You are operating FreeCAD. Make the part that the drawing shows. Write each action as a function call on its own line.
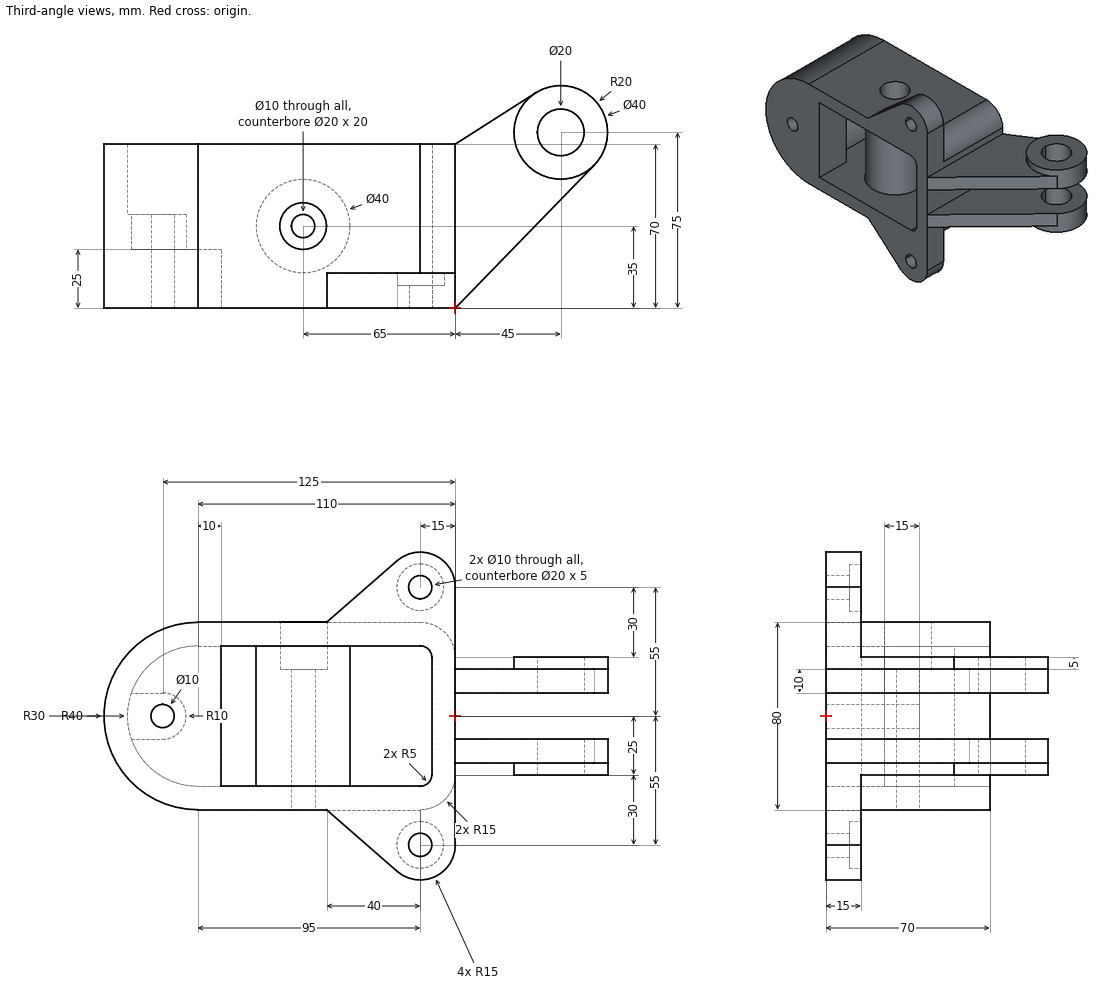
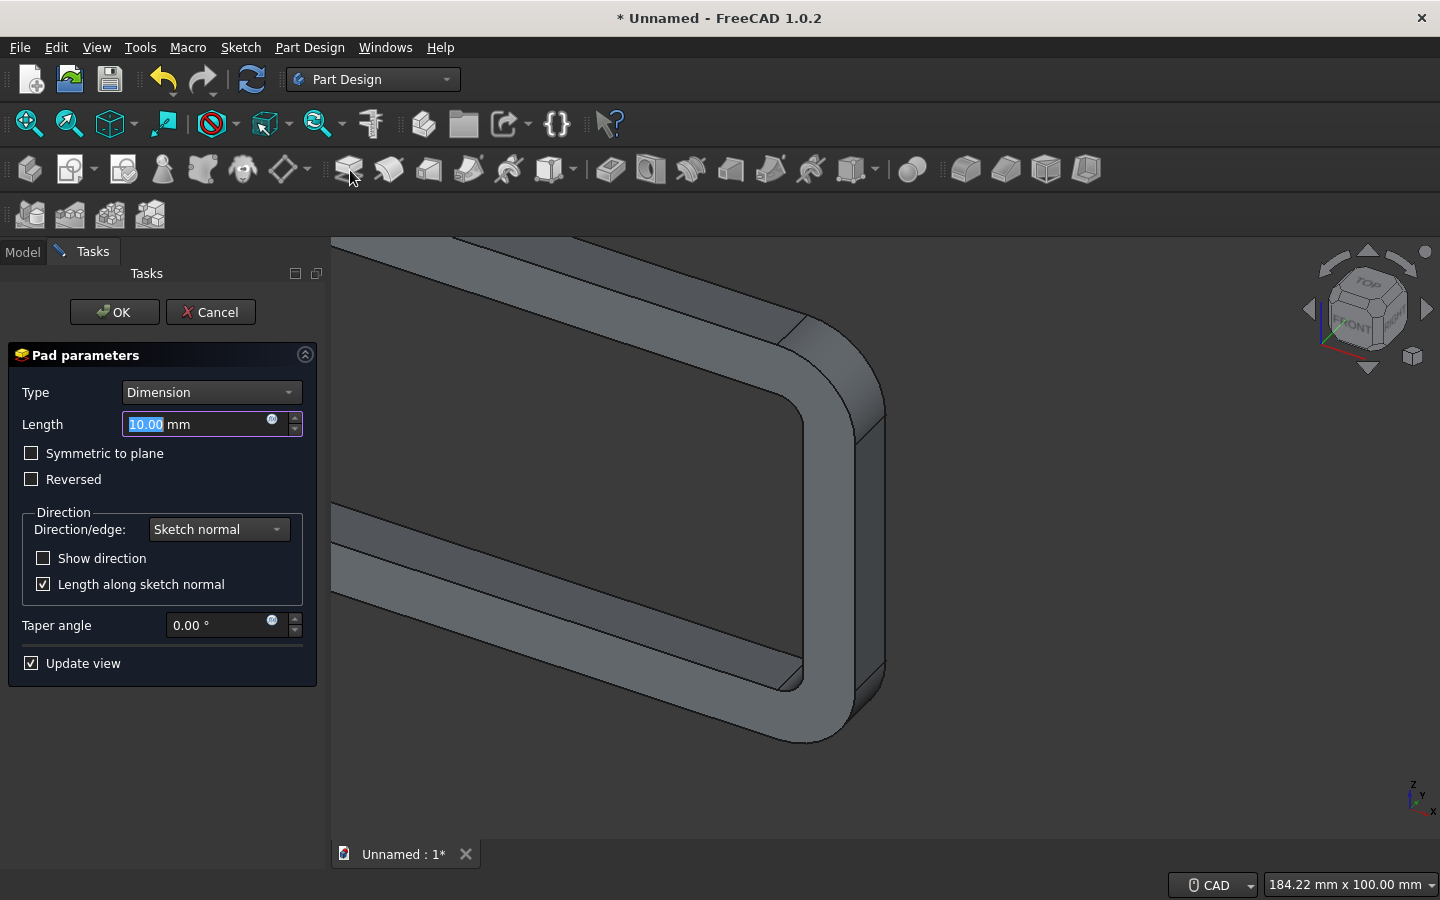
text(70)
key(Tab)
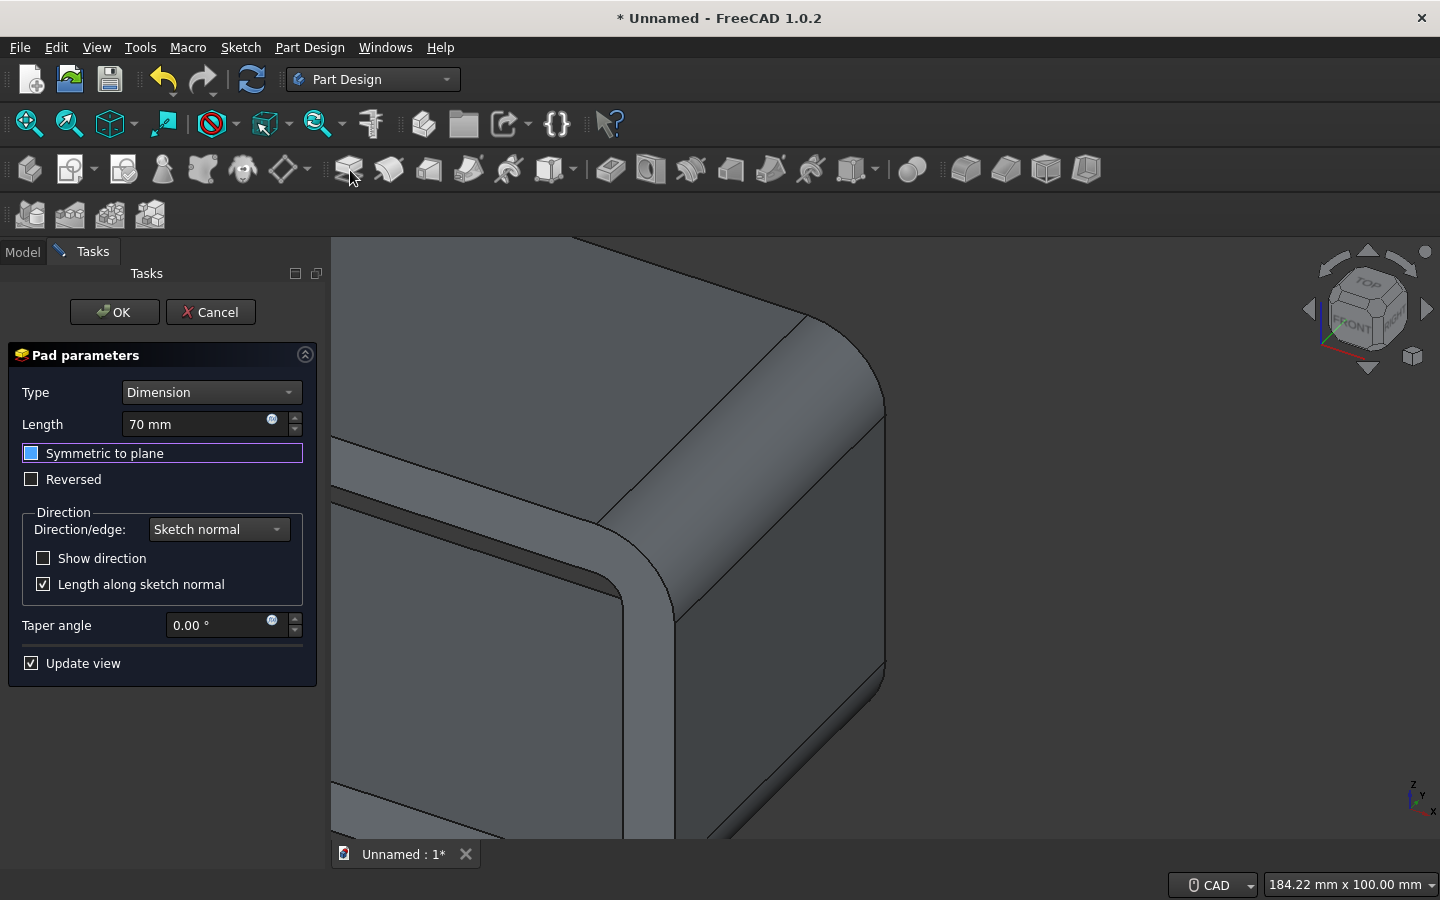
click(30, 479)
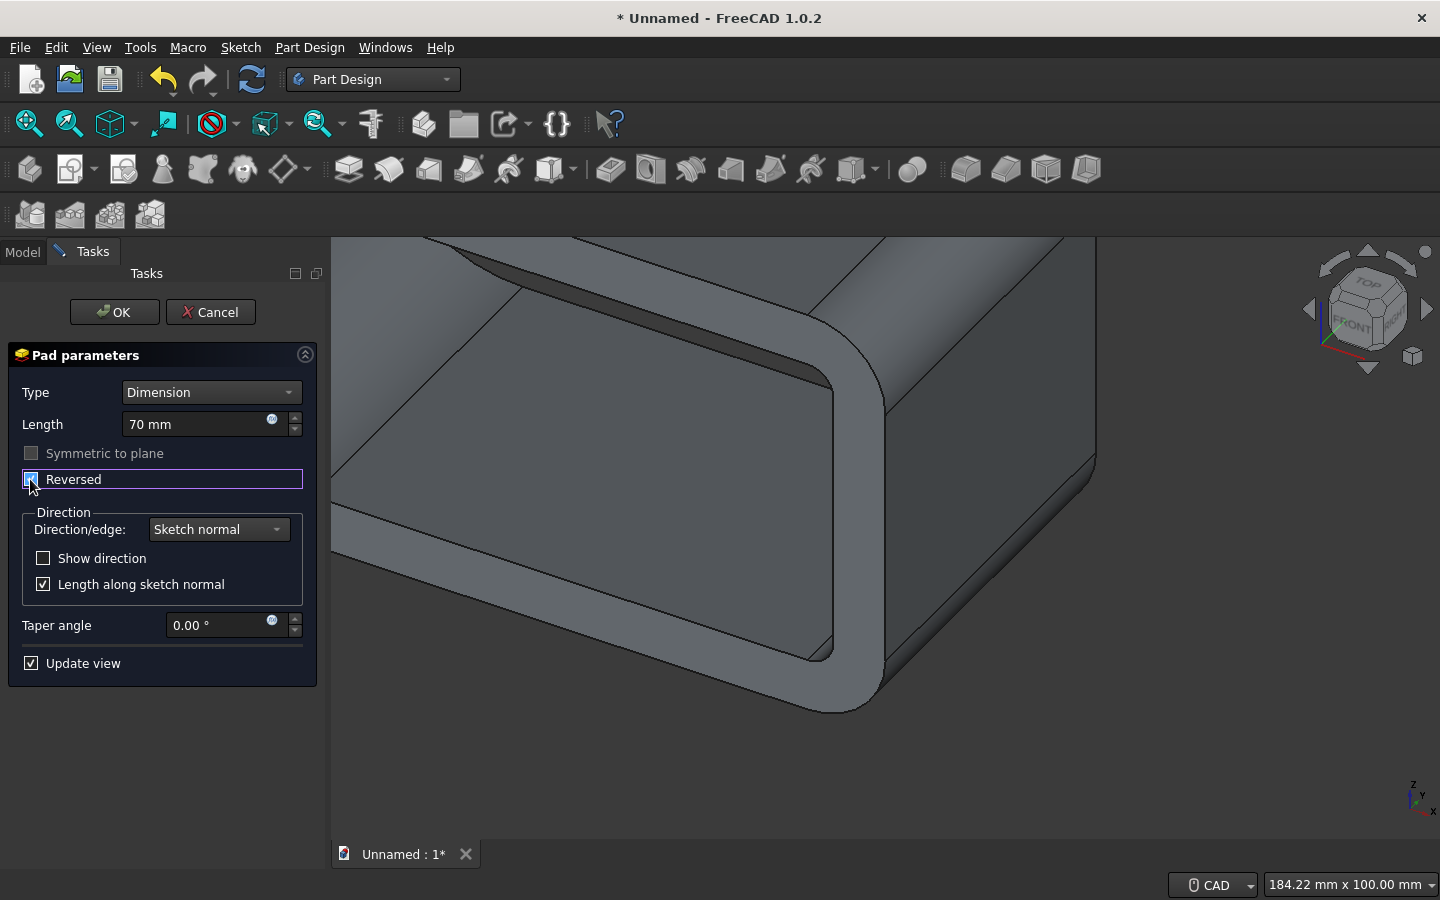
click(115, 312)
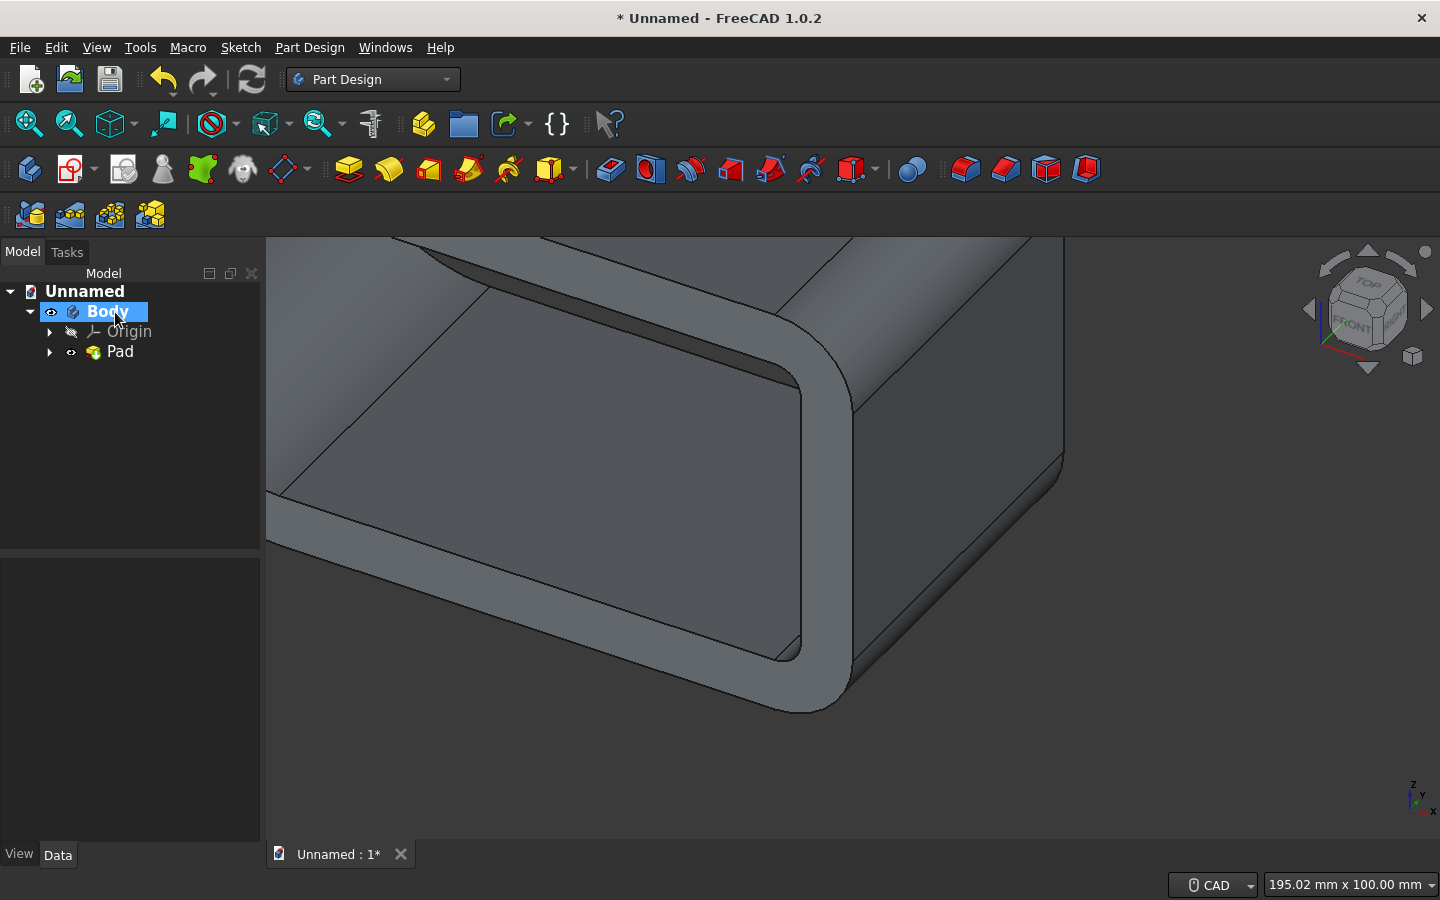
key(v)
key(f)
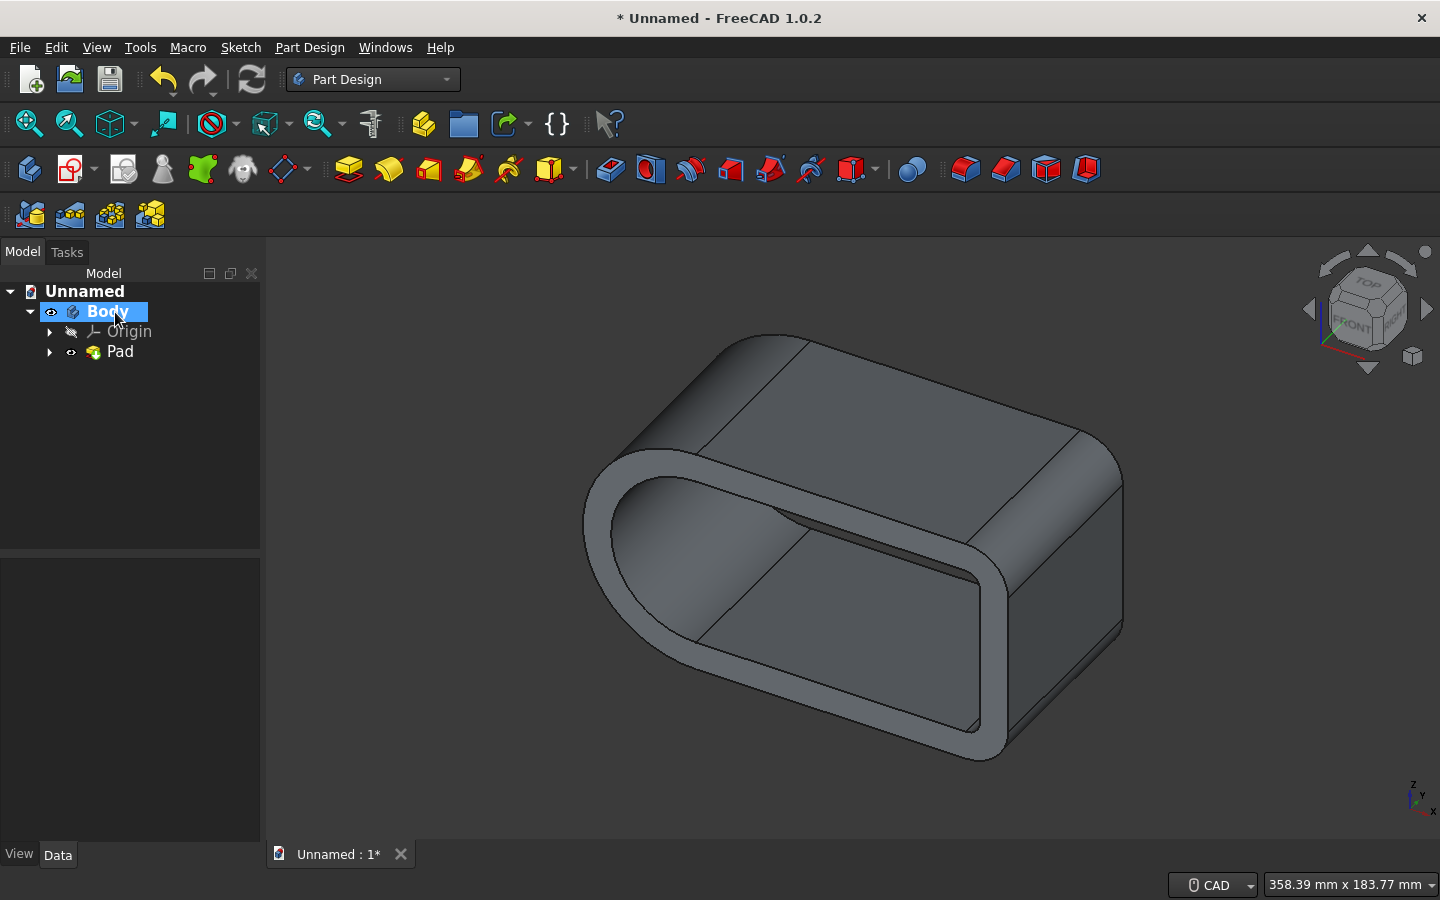
click(674, 646)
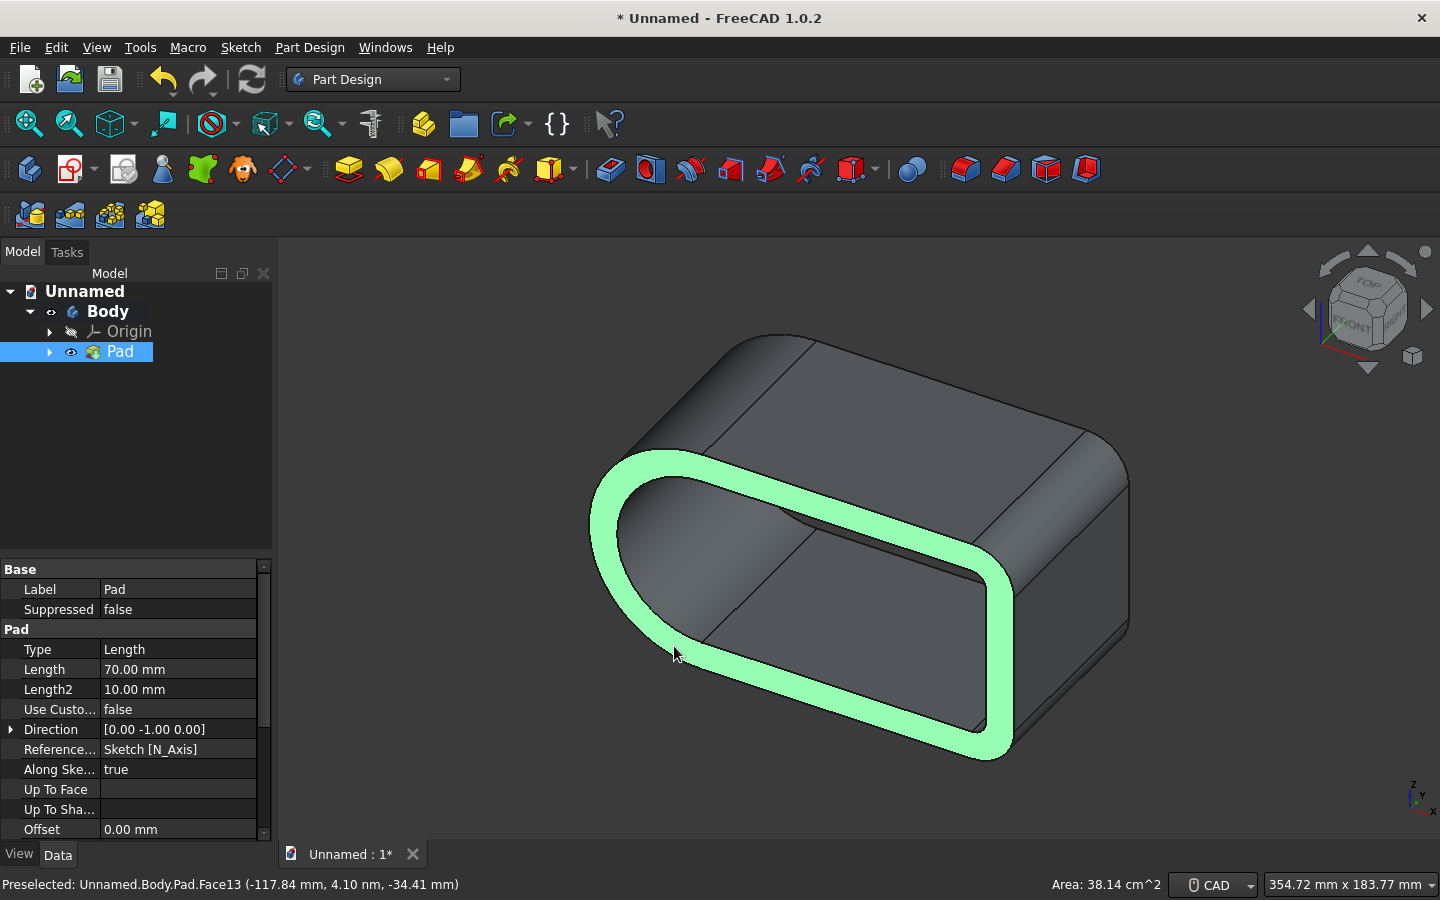
click(70, 170)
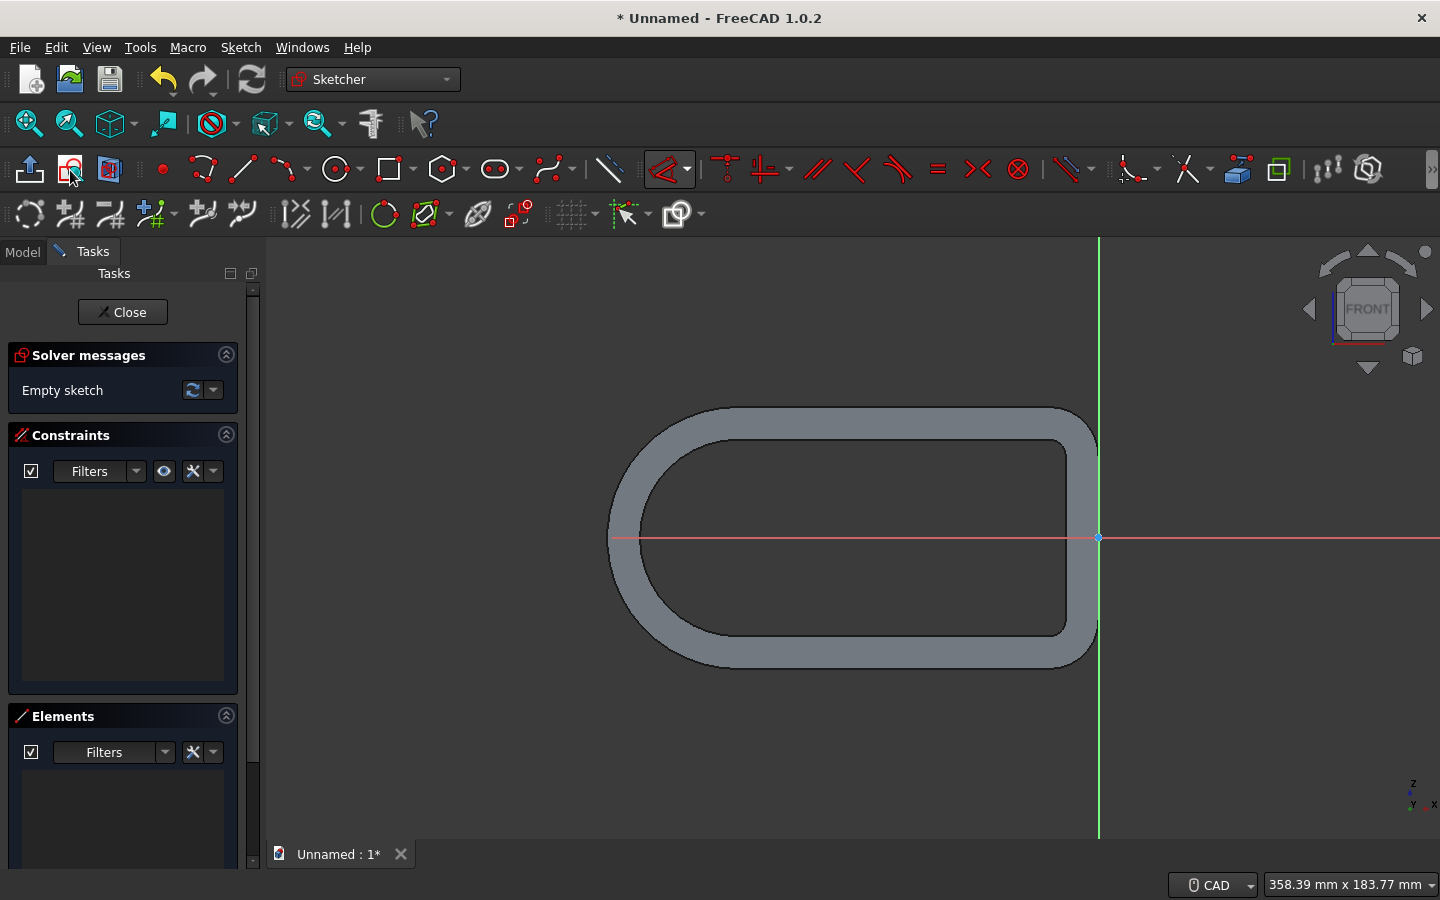
scroll(1041, 538, up, 2)